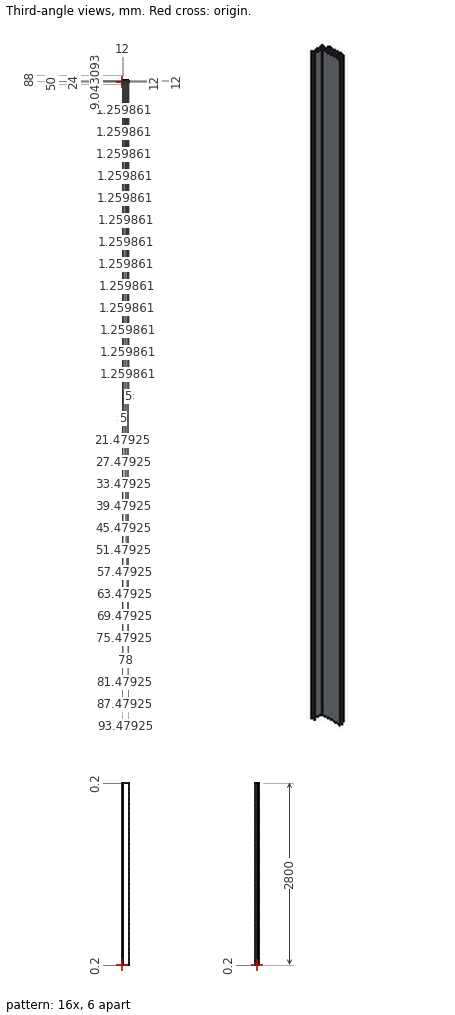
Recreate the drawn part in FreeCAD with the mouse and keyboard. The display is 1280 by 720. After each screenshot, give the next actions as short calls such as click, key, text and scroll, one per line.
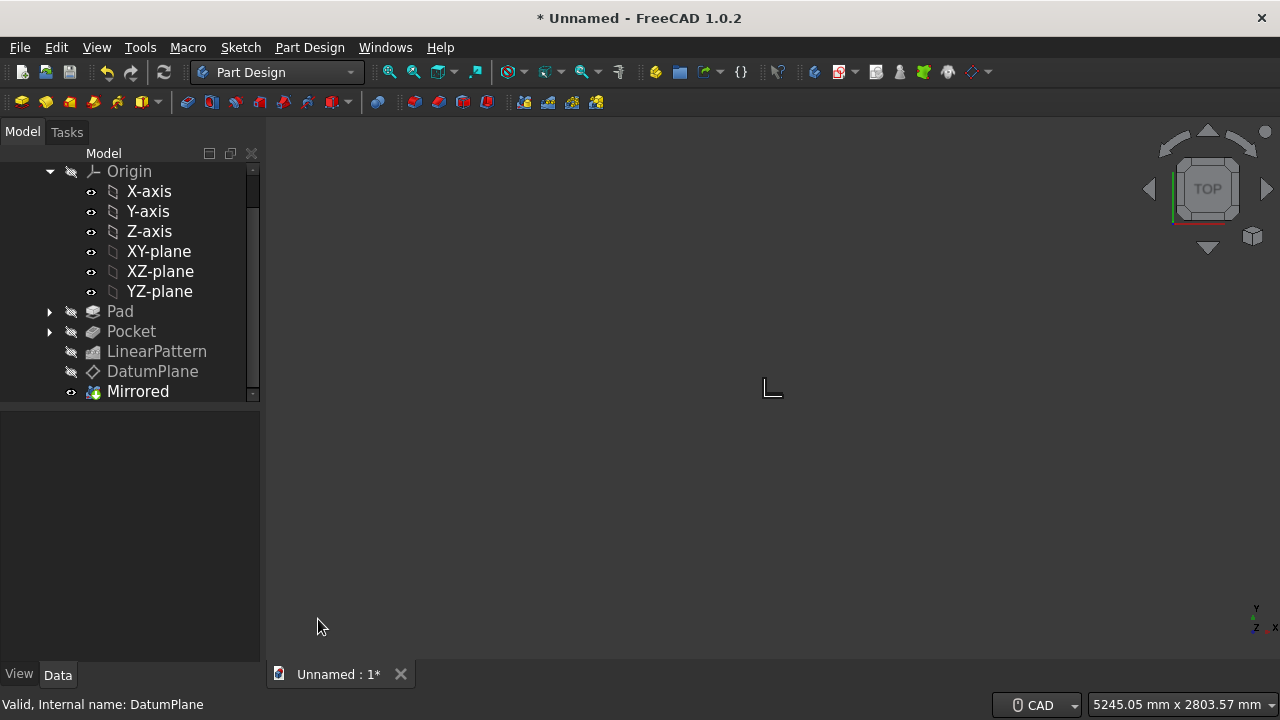
click(840, 72)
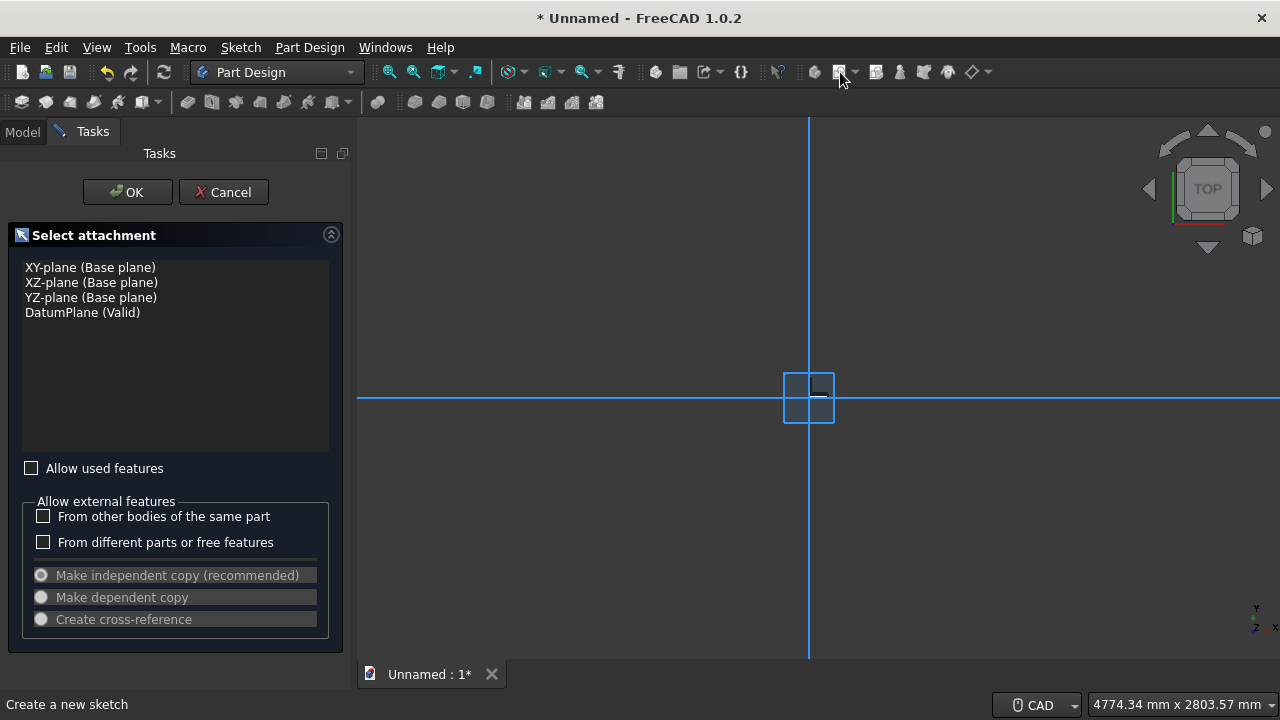
click(82, 268)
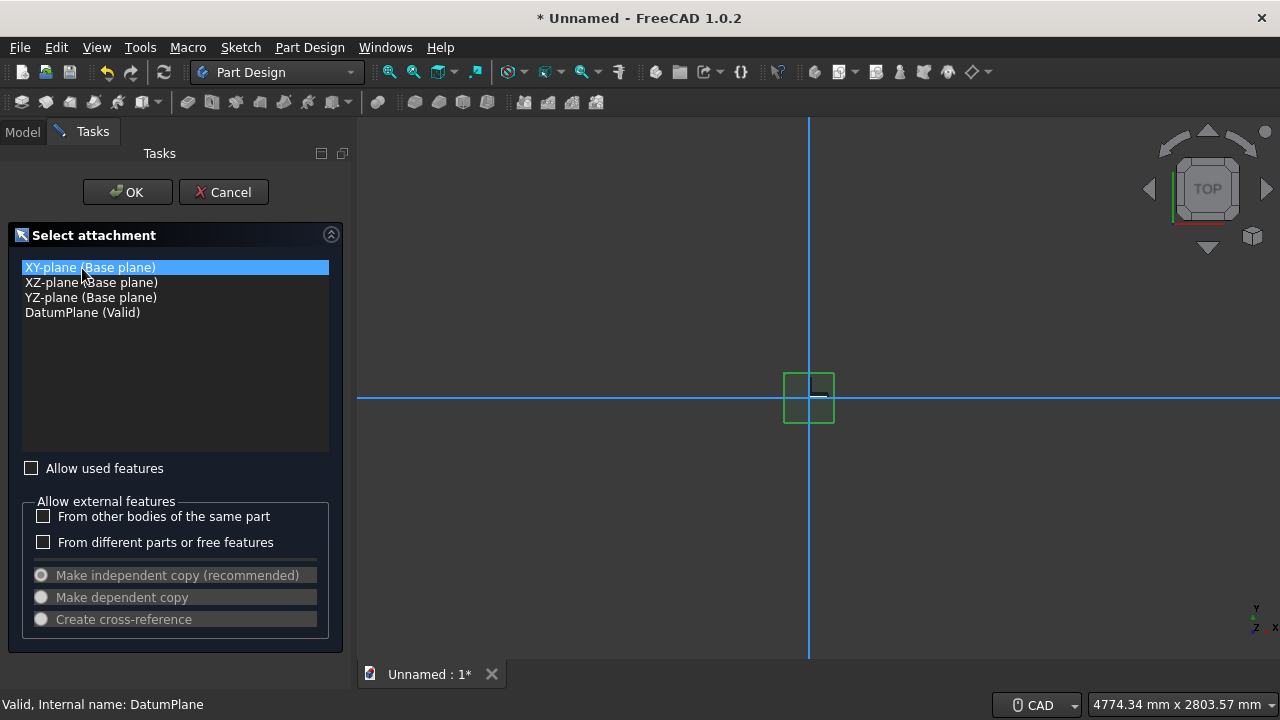
click(128, 192)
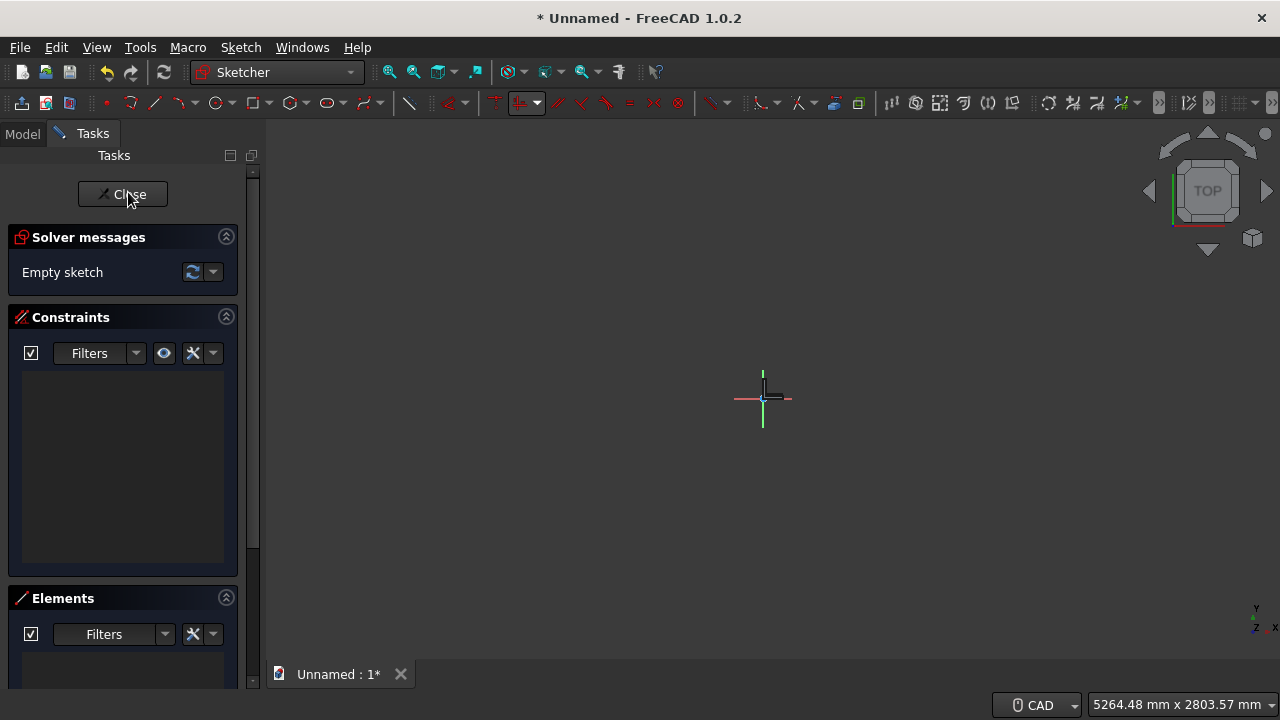
click(70, 104)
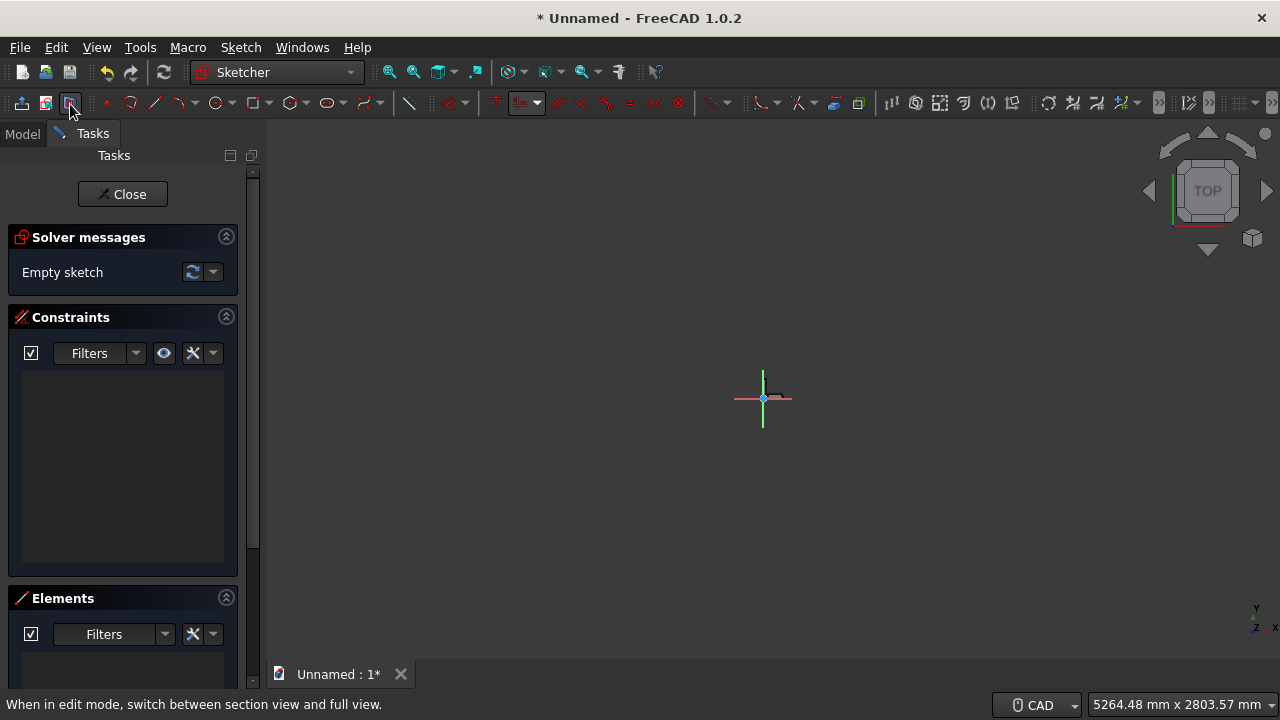
scroll(772, 395, up, 15)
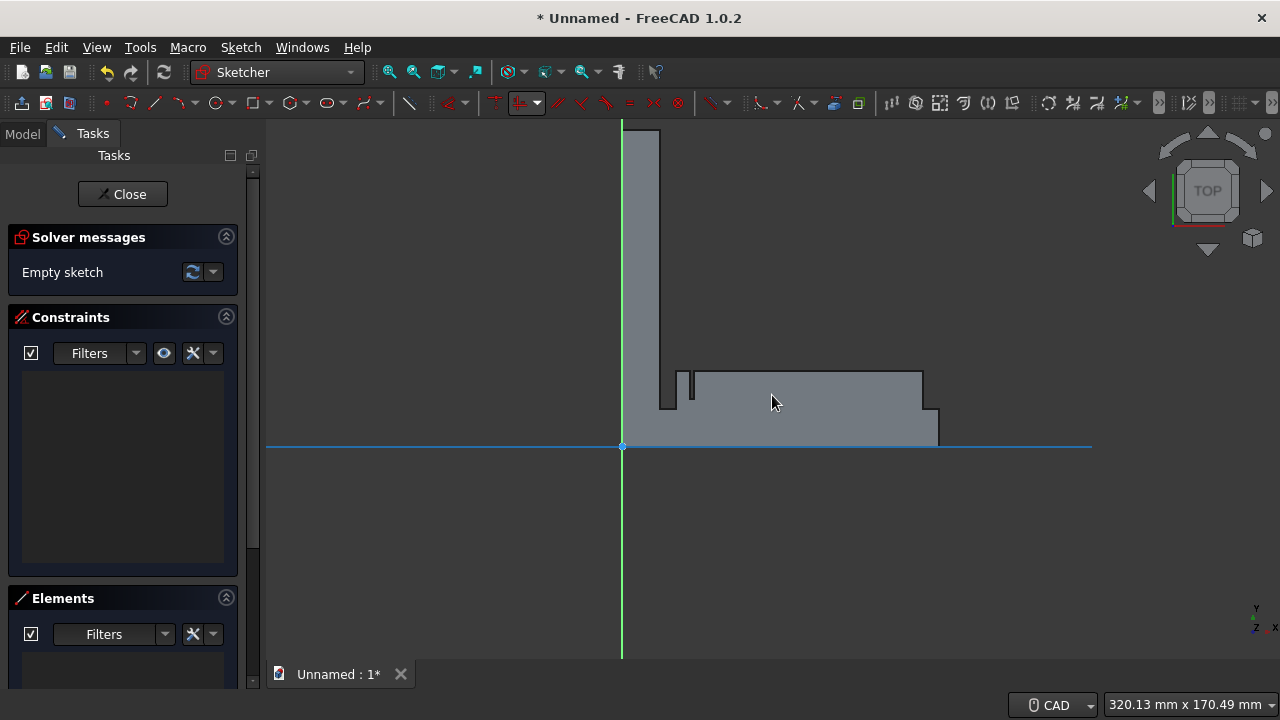
scroll(697, 382, up, 11)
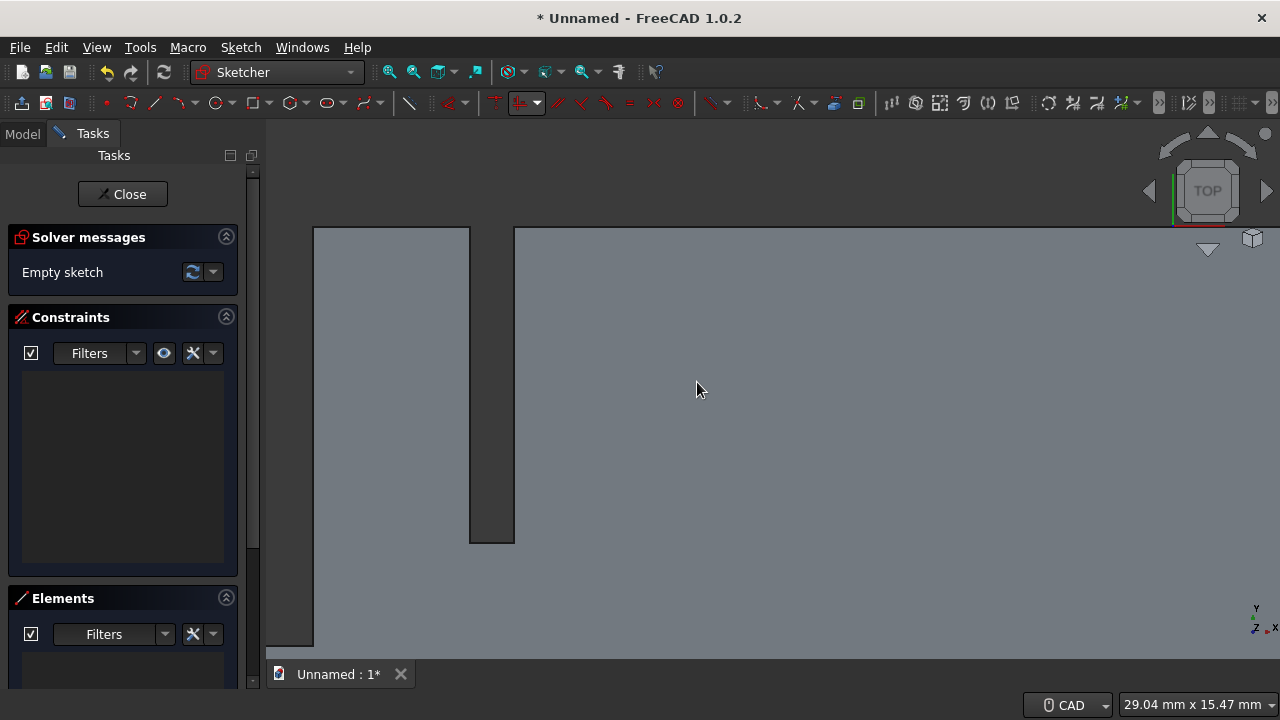
click(254, 104)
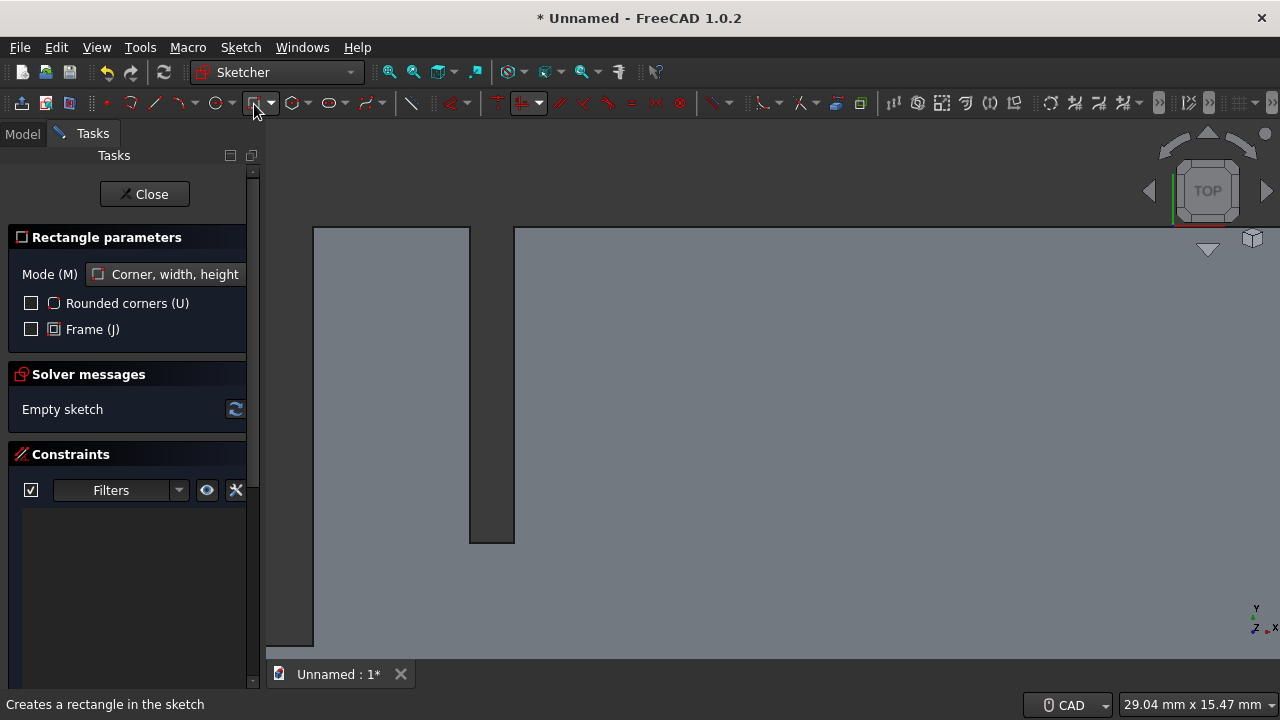
click(679, 227)
move(723, 543)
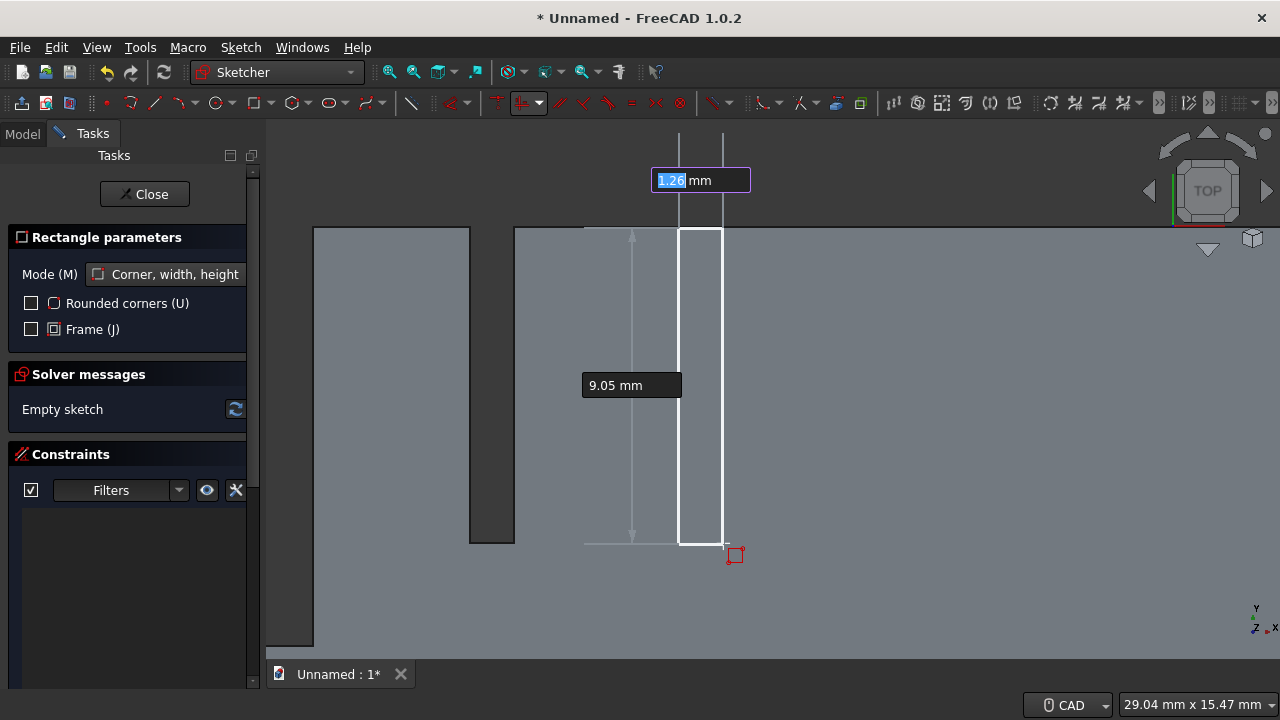
text(1.259861)
key(Tab)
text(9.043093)
key(Return)
key(Escape)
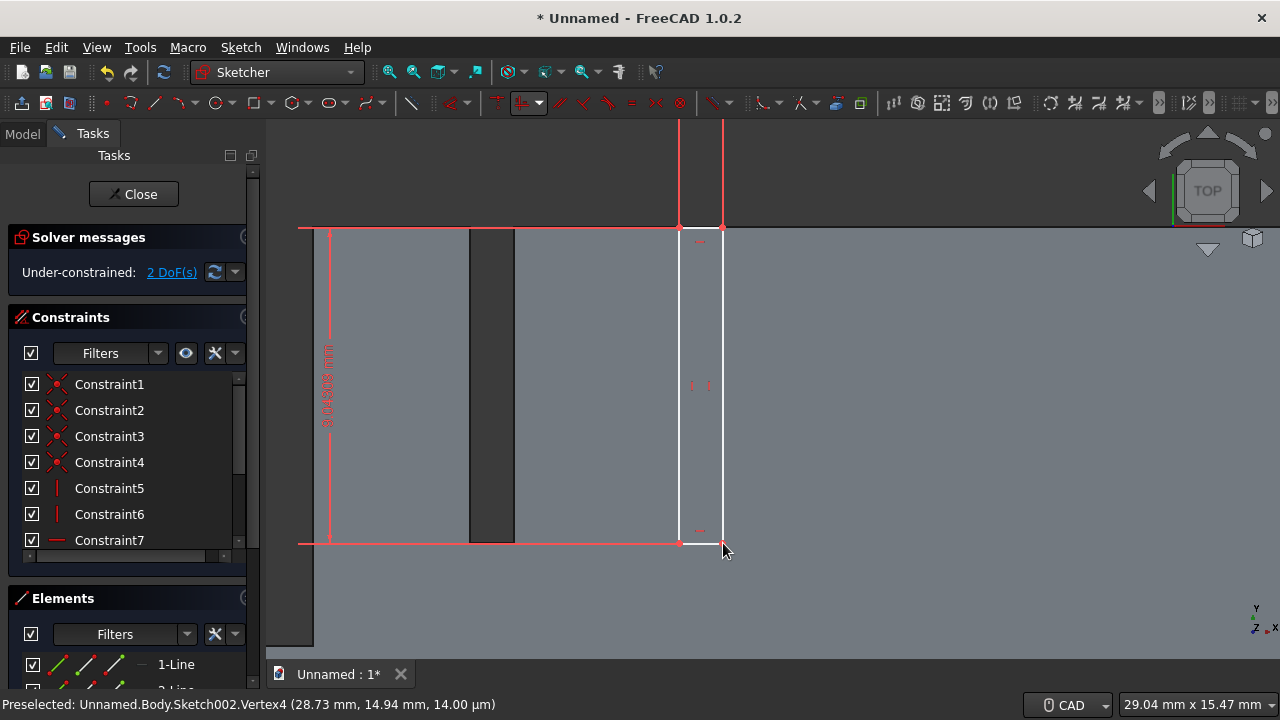
click(450, 104)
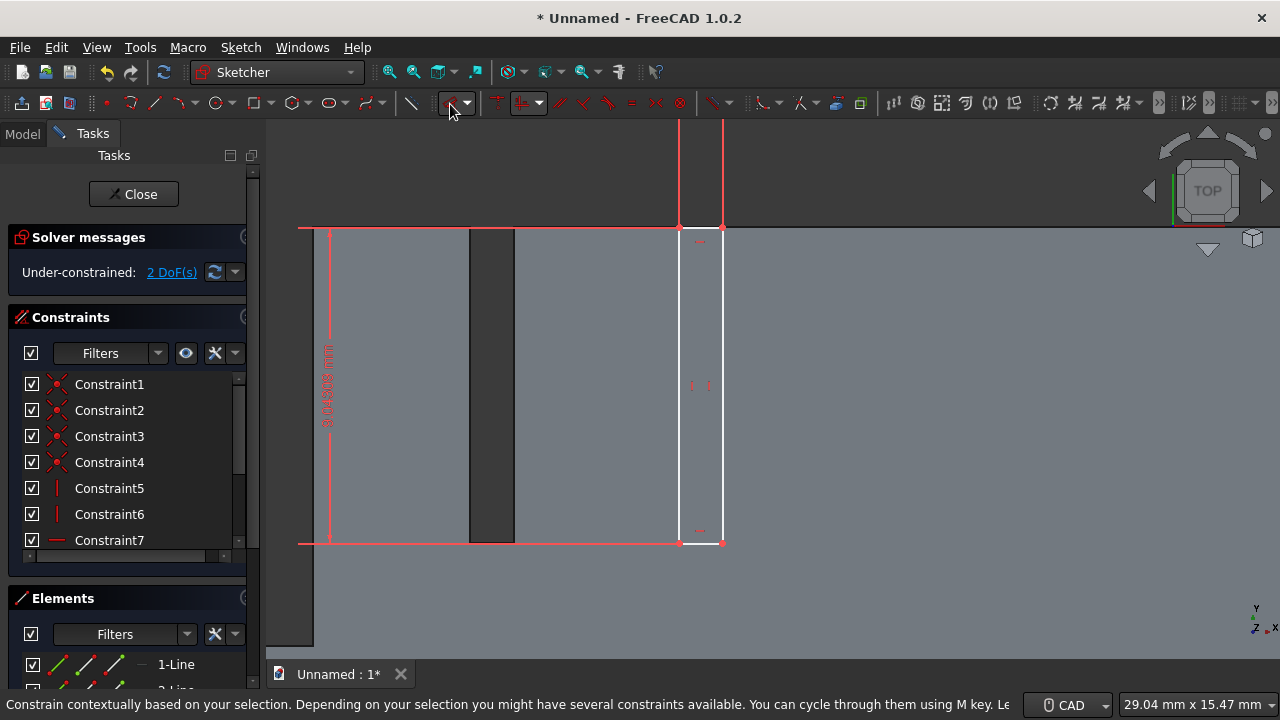
click(679, 228)
click(713, 571)